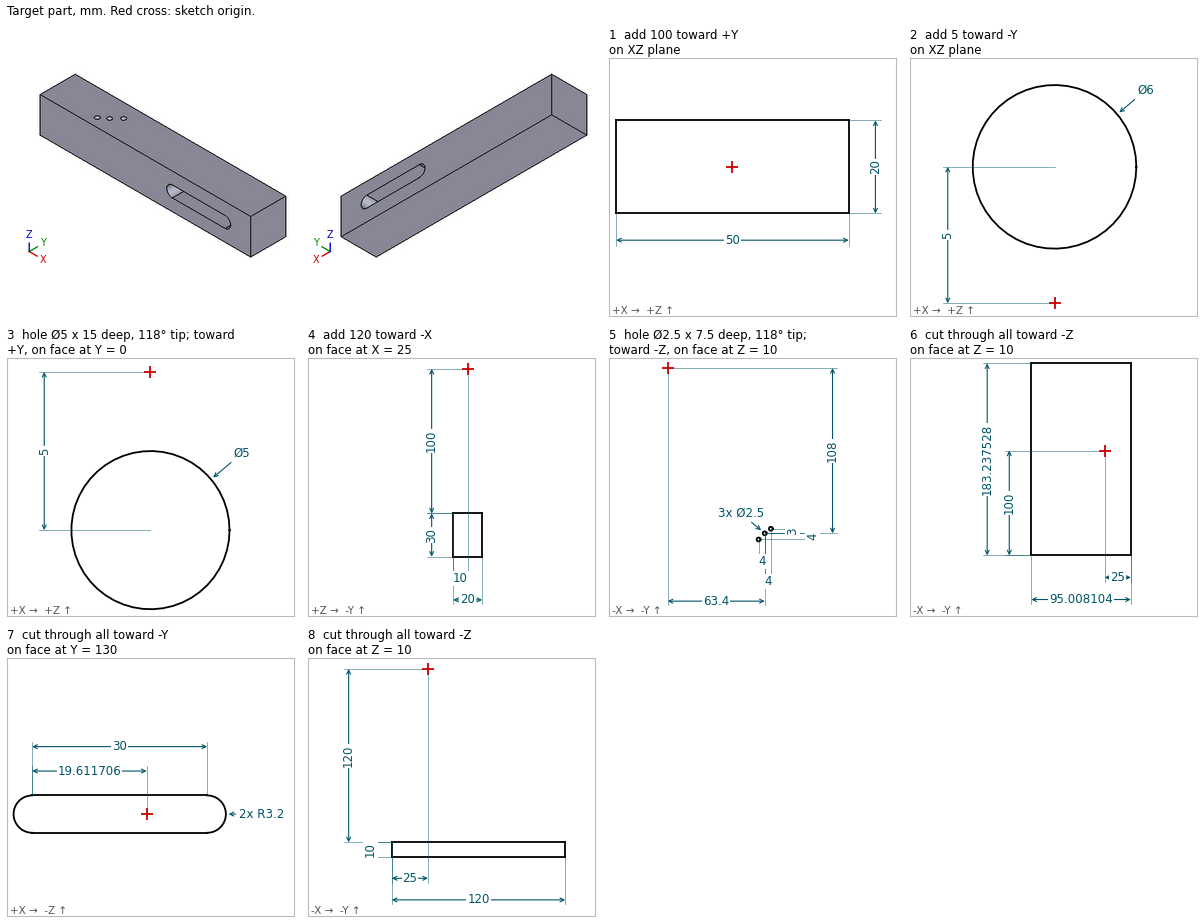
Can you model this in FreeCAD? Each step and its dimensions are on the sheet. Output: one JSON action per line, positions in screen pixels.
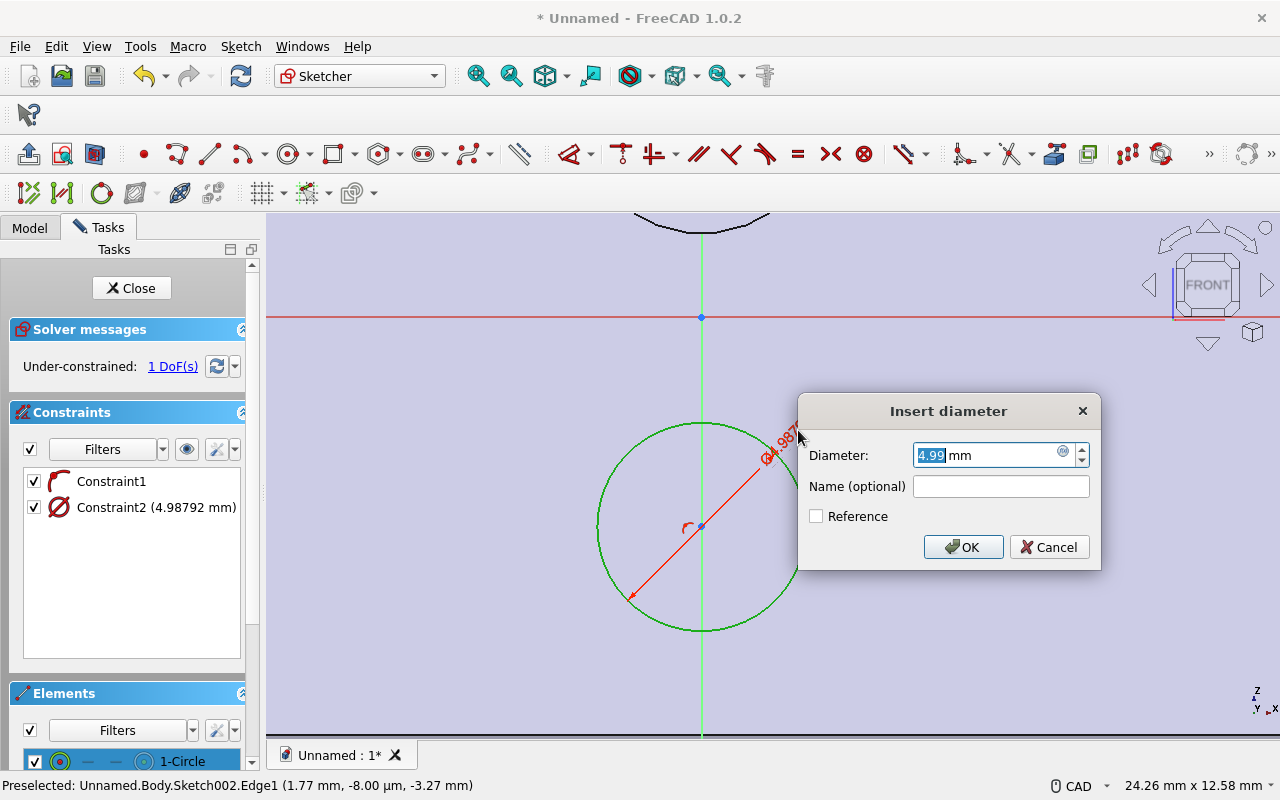
{"action": "type", "text": "5"}
{"action": "key", "text": "Return"}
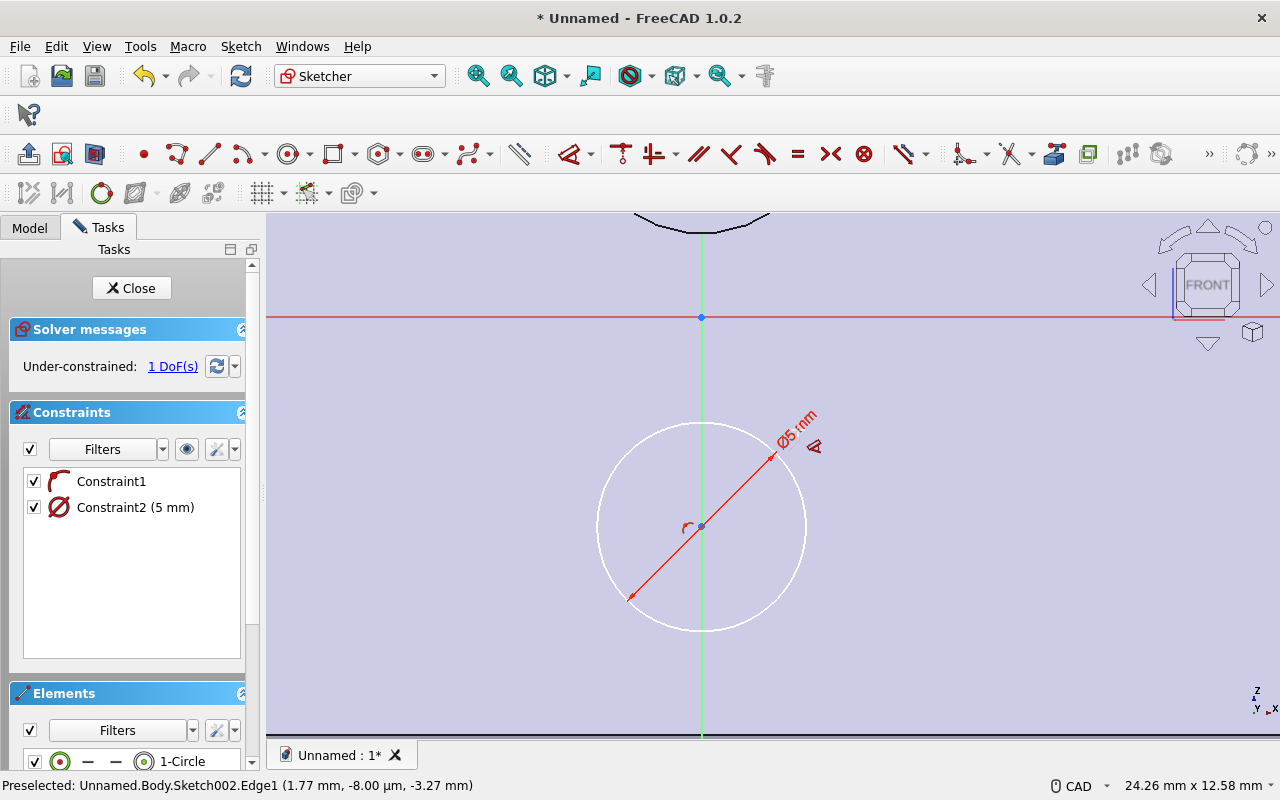
{"action": "left_click", "coordinate": [702, 527]}
{"action": "left_click", "coordinate": [736, 374]}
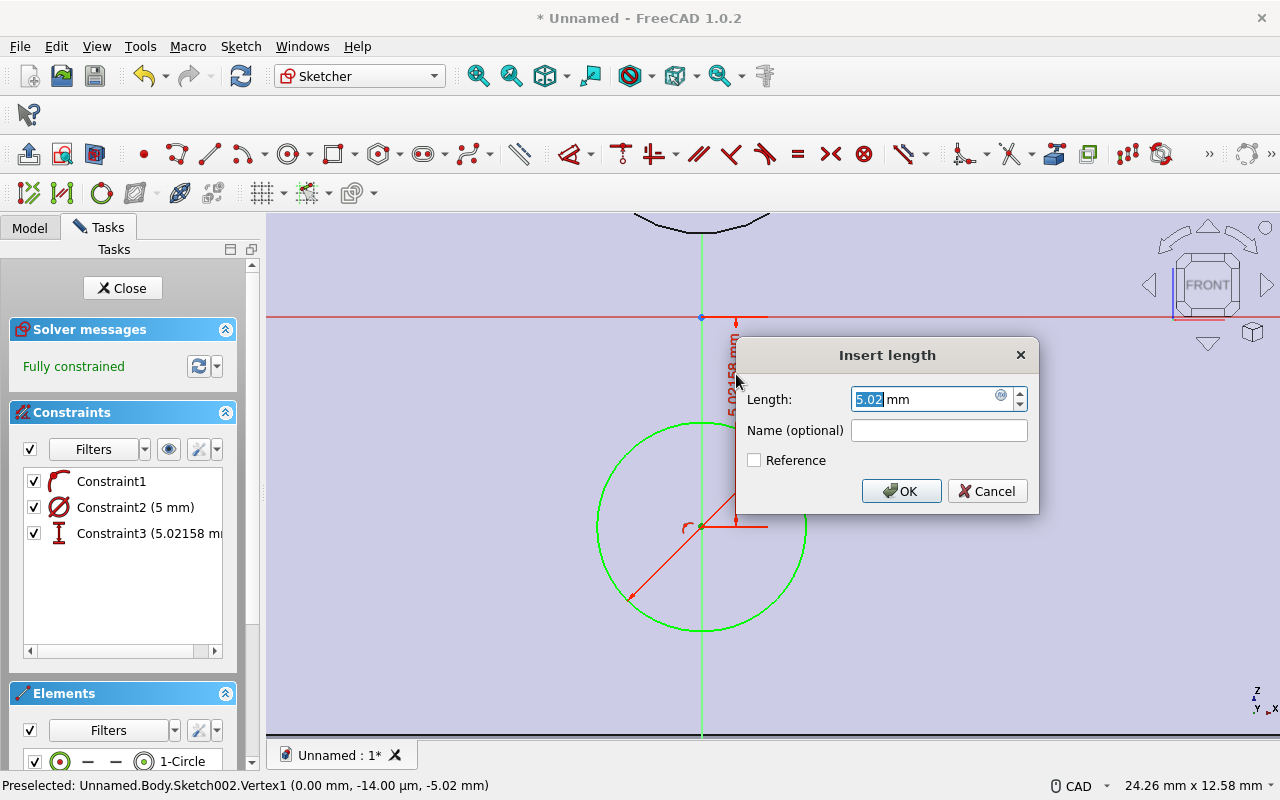
{"action": "type", "text": "5"}
{"action": "key", "text": "Return"}
{"action": "key", "text": "Escape"}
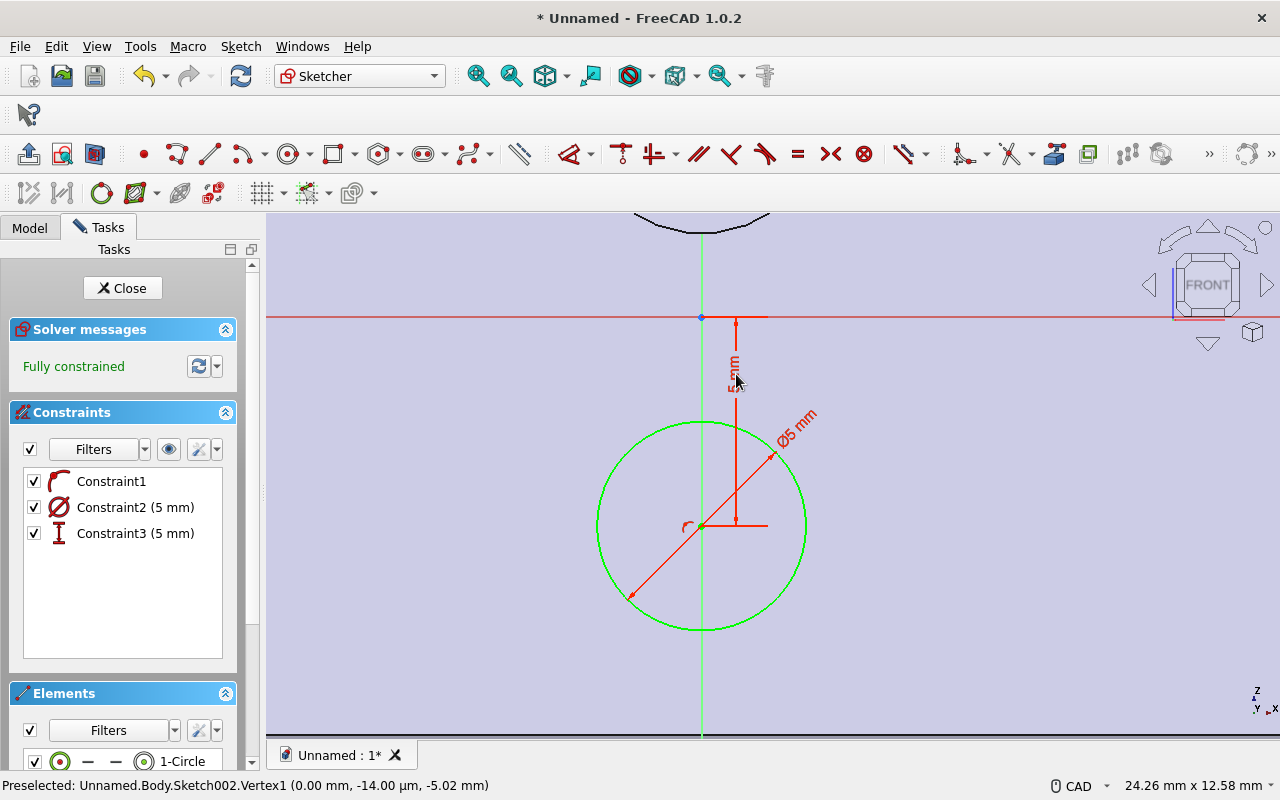
{"action": "left_click", "coordinate": [123, 288]}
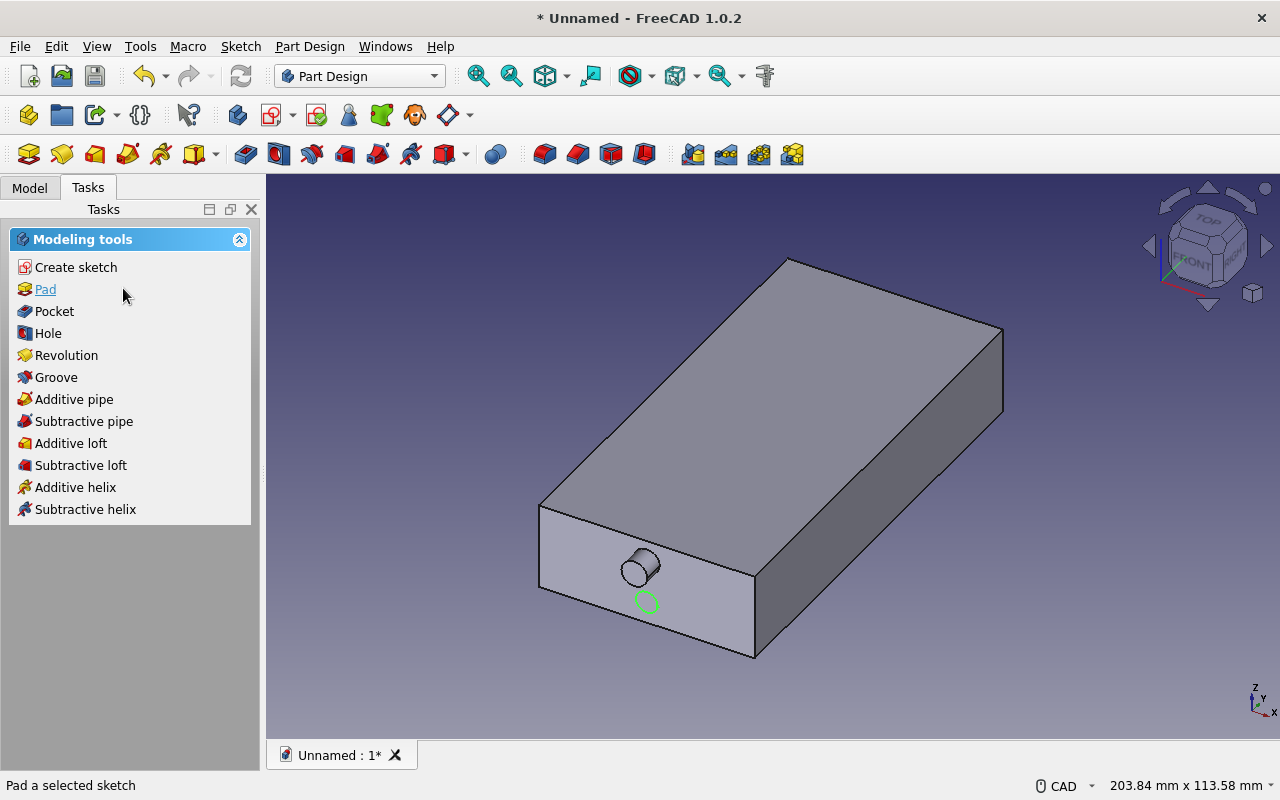
{"action": "left_click", "coordinate": [279, 154]}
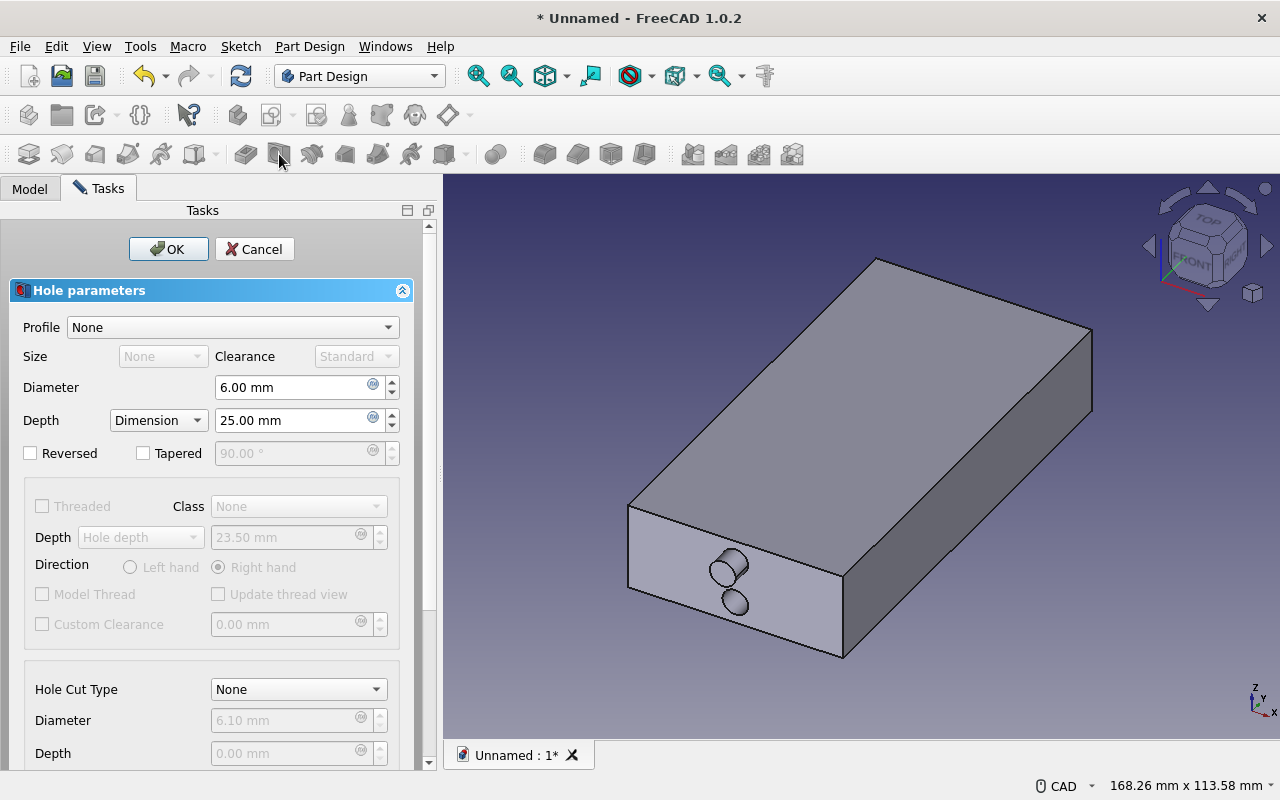
{"action": "triple_click", "coordinate": [300, 388]}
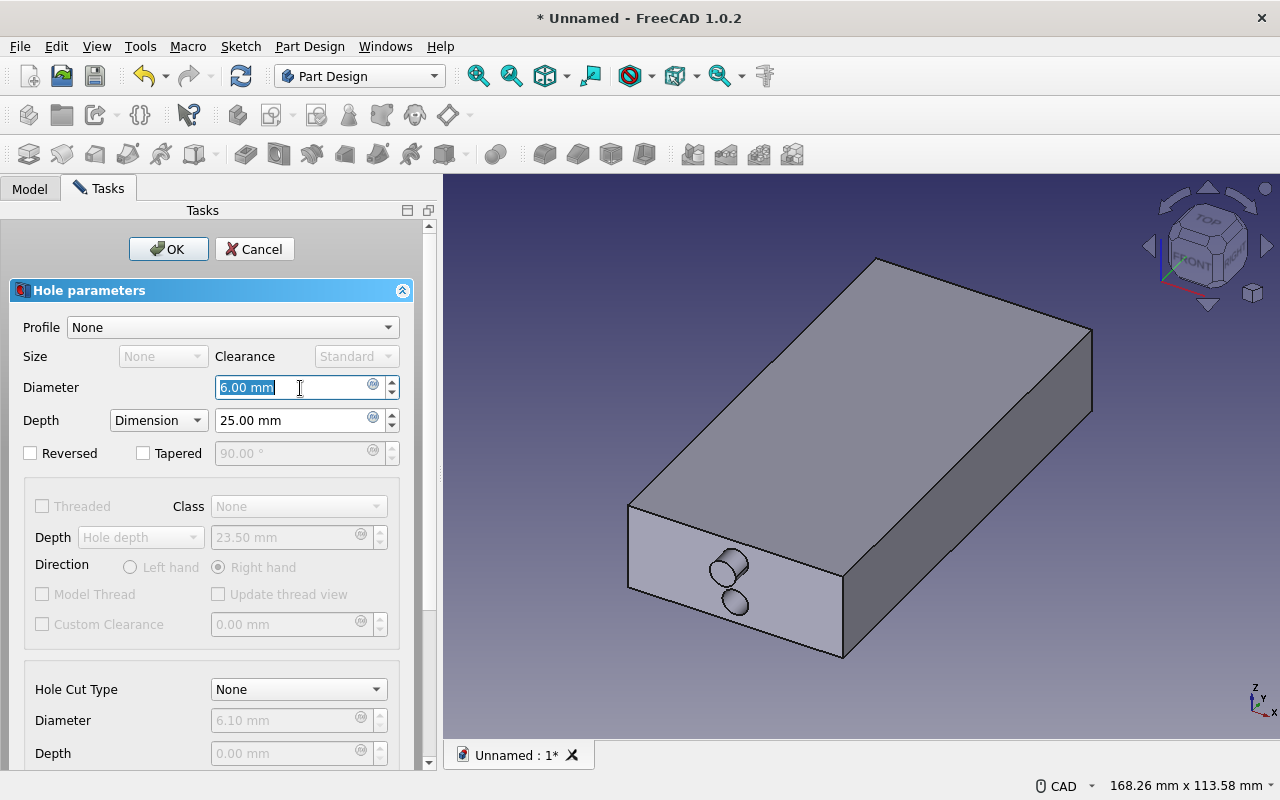
{"action": "type", "text": "5"}
{"action": "key", "text": "Tab"}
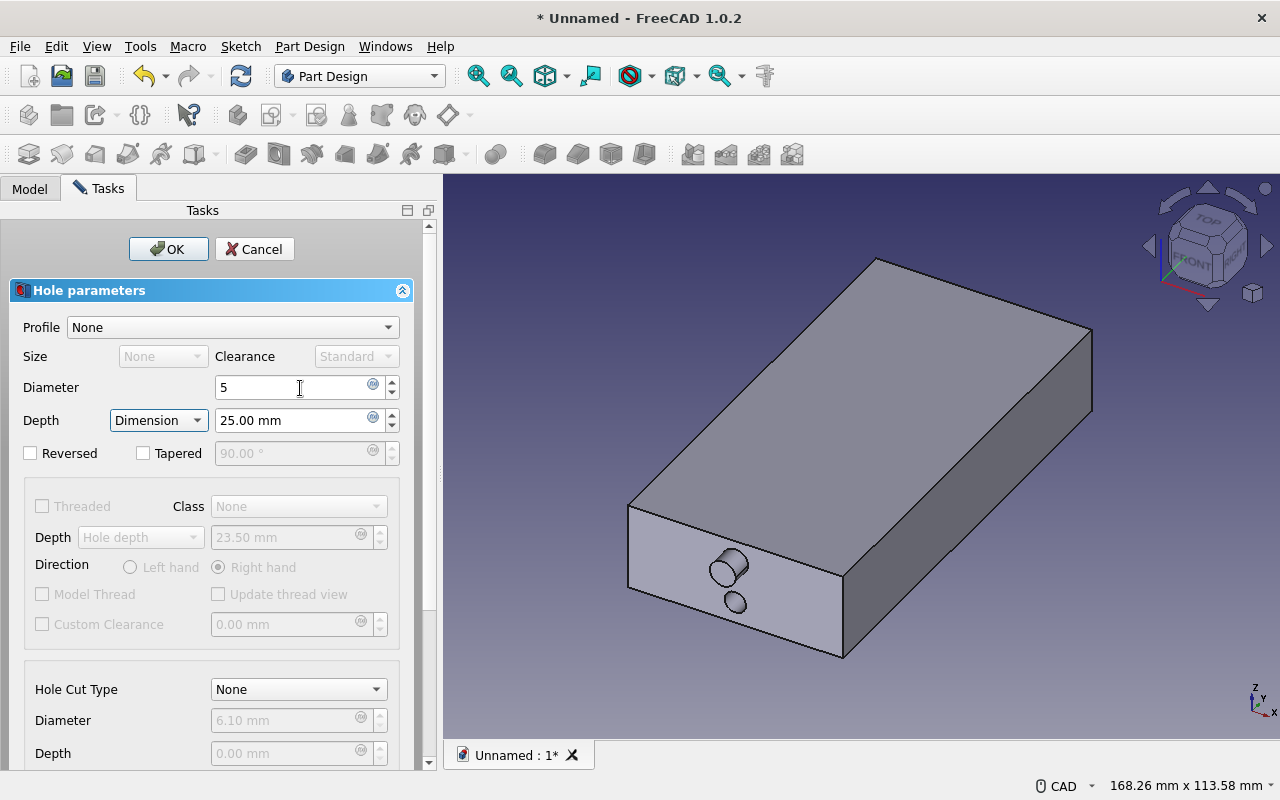
{"action": "triple_click", "coordinate": [300, 420]}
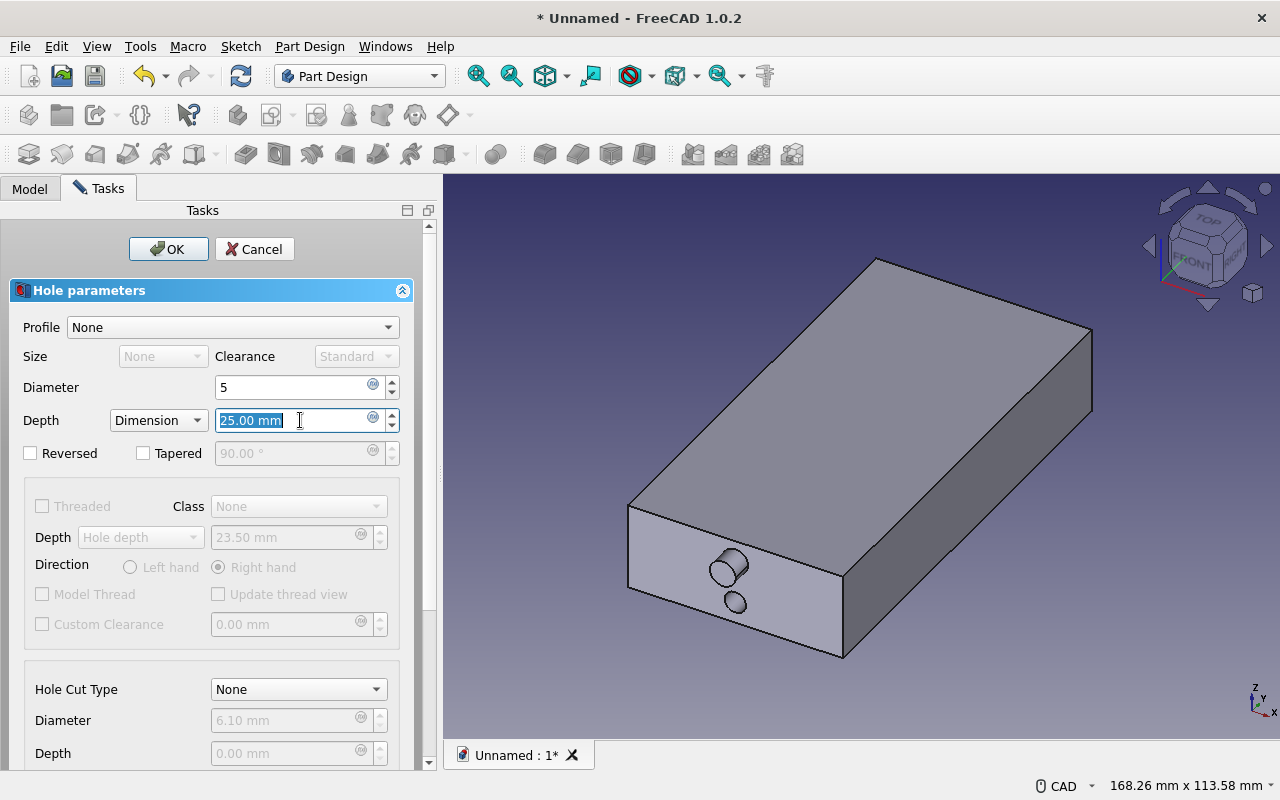
{"action": "type", "text": "15"}
{"action": "key", "text": "Tab"}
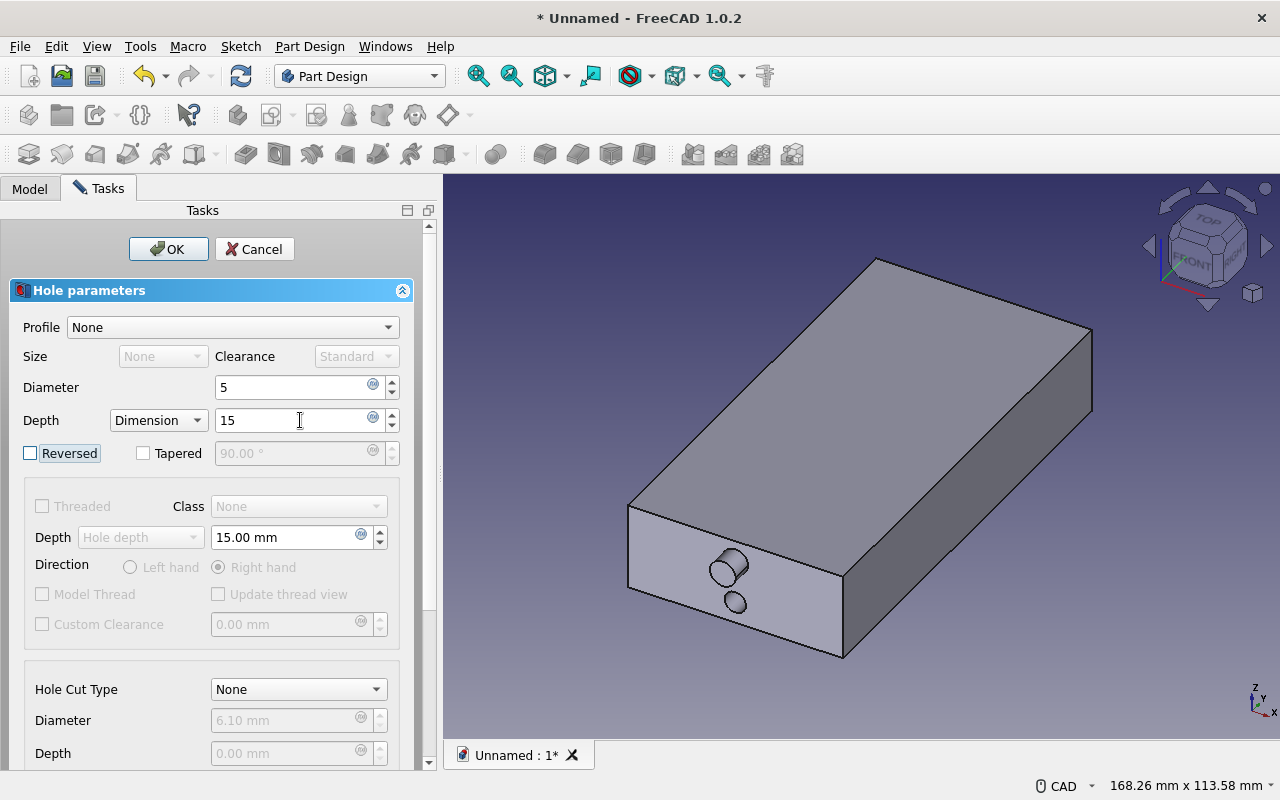
{"action": "left_click", "coordinate": [169, 249]}